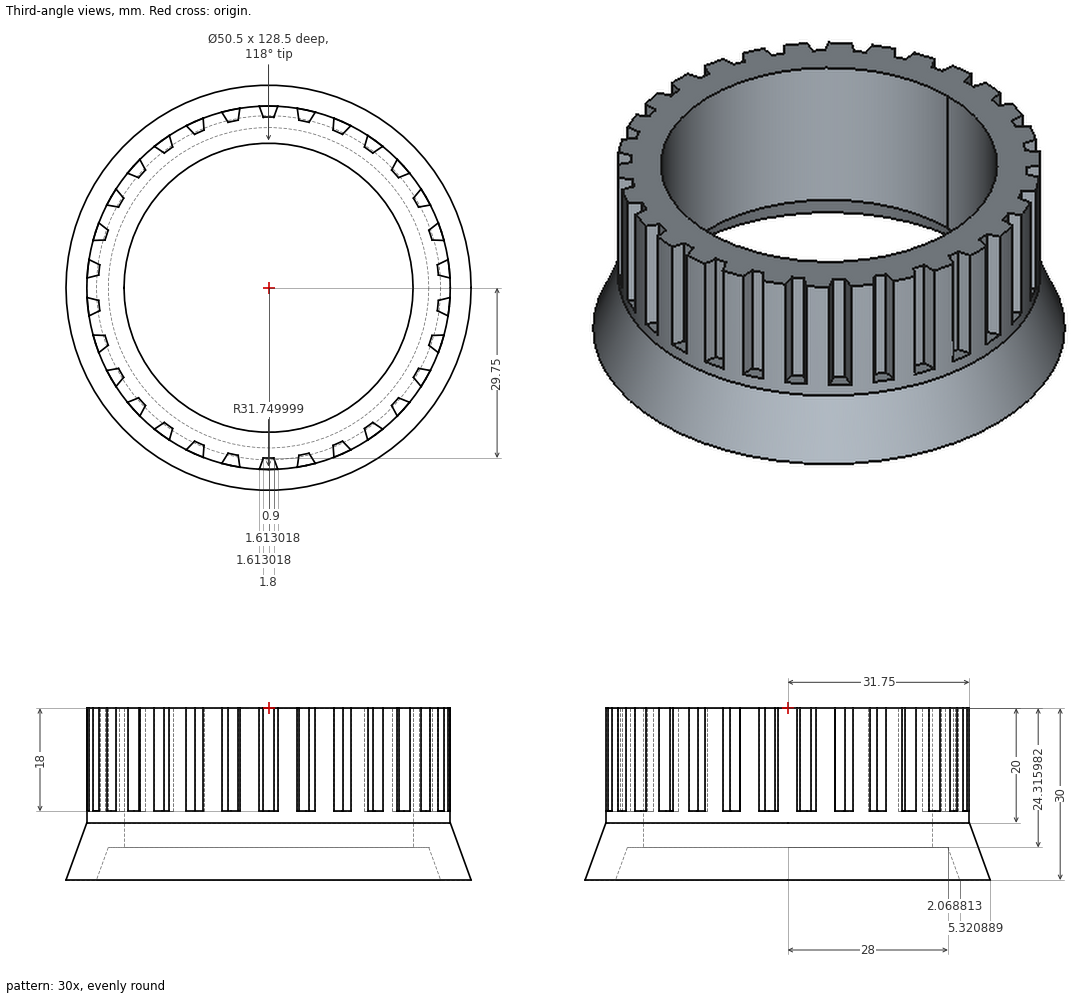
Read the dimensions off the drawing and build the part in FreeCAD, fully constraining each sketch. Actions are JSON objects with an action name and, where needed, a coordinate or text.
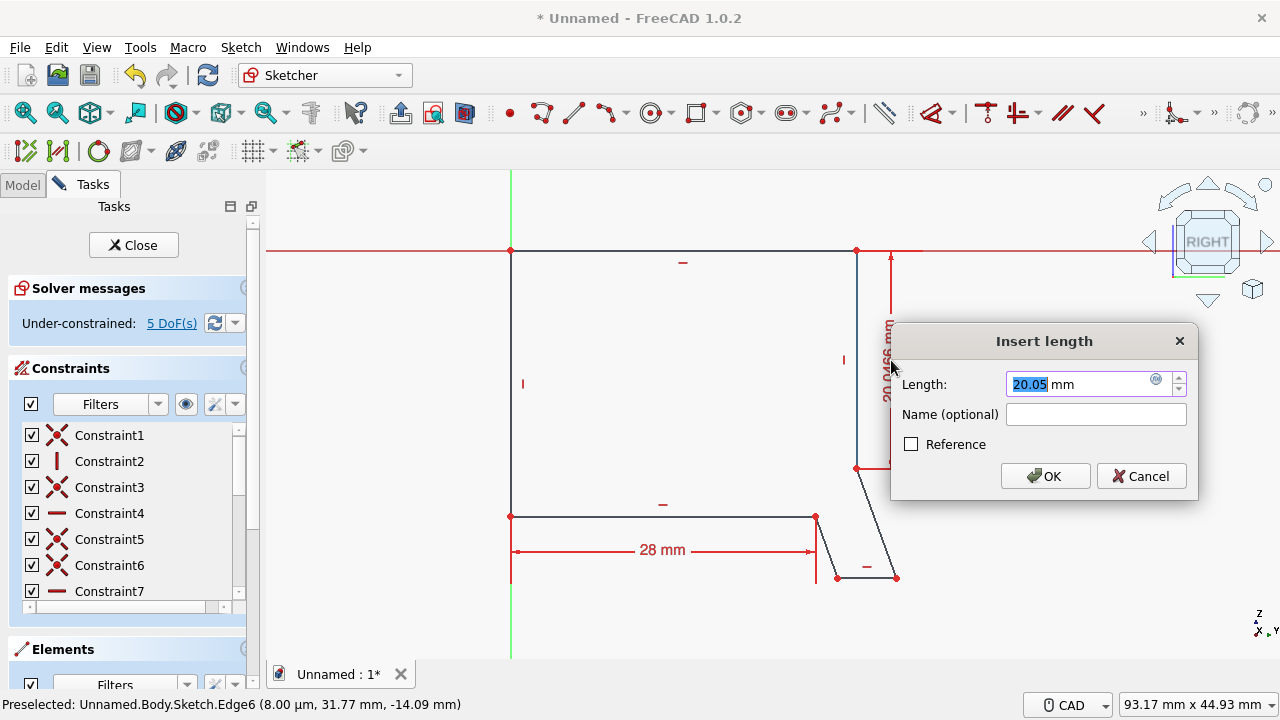
{"action": "type", "text": "20"}
{"action": "key", "text": "Return"}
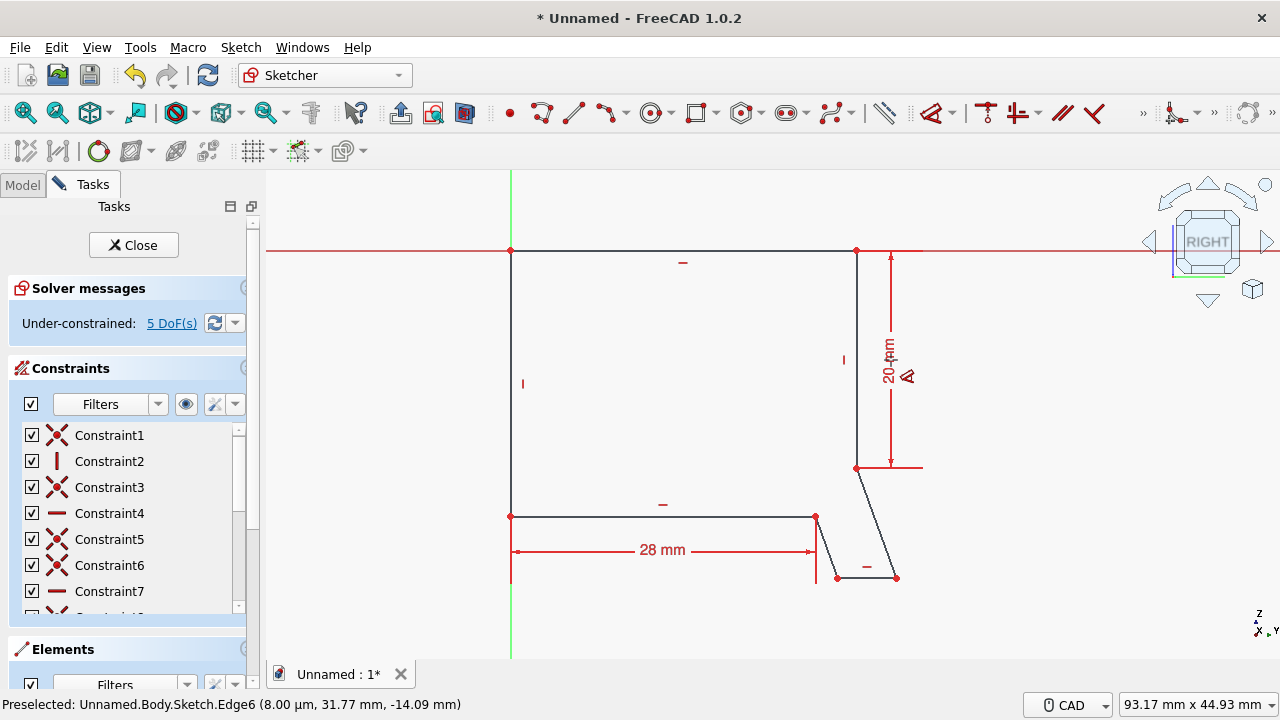
{"action": "left_click", "coordinate": [838, 578]}
{"action": "left_click", "coordinate": [477, 414]}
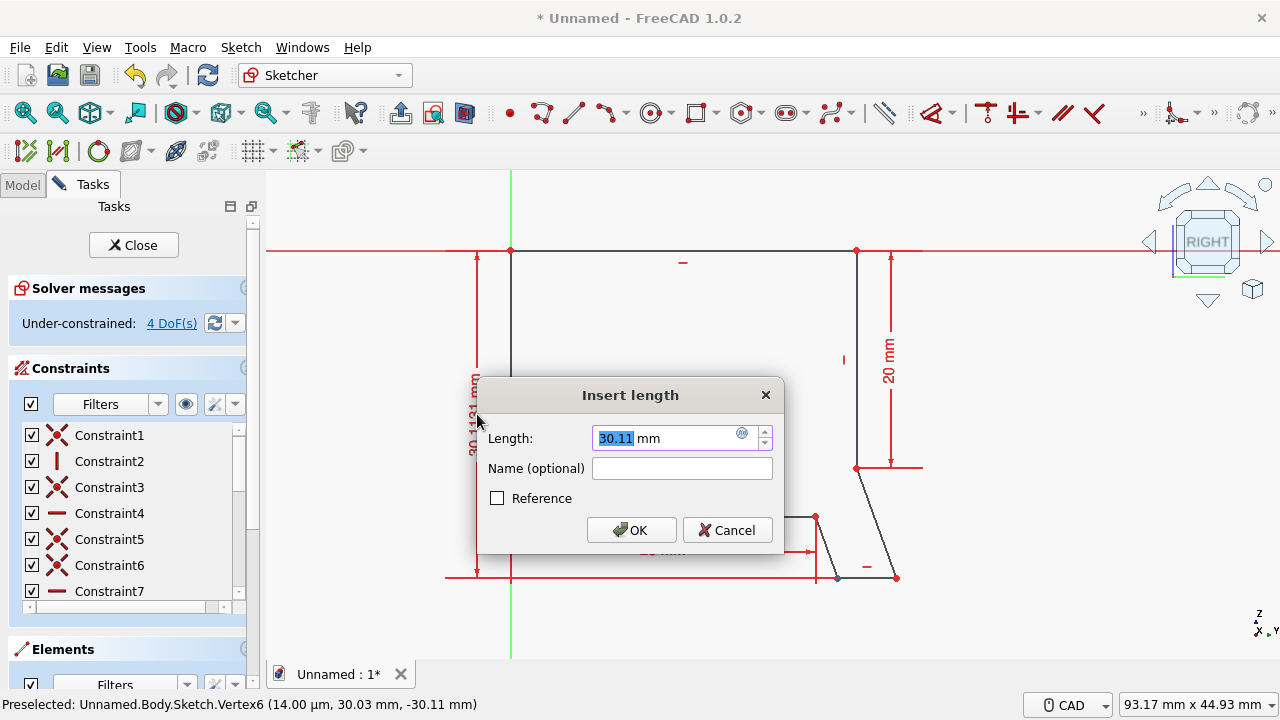
{"action": "type", "text": "30"}
{"action": "key", "text": "Return"}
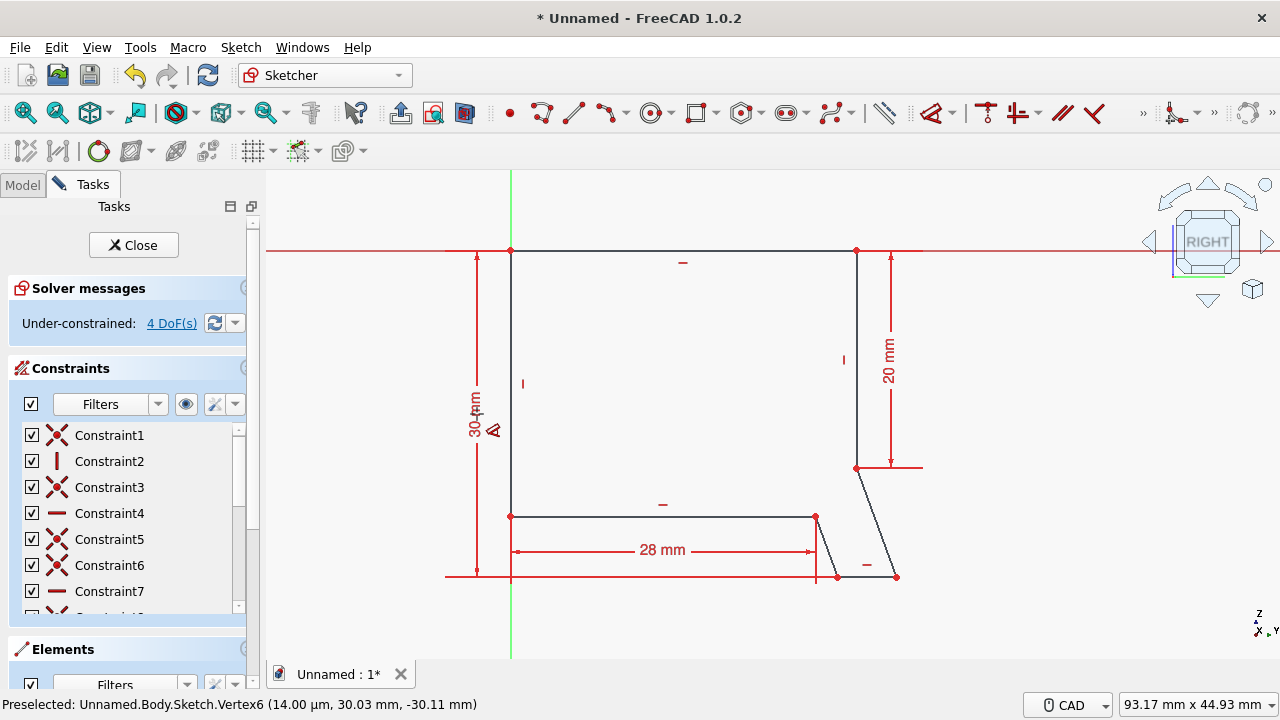
{"action": "left_click", "coordinate": [753, 251]}
{"action": "left_click", "coordinate": [684, 217]}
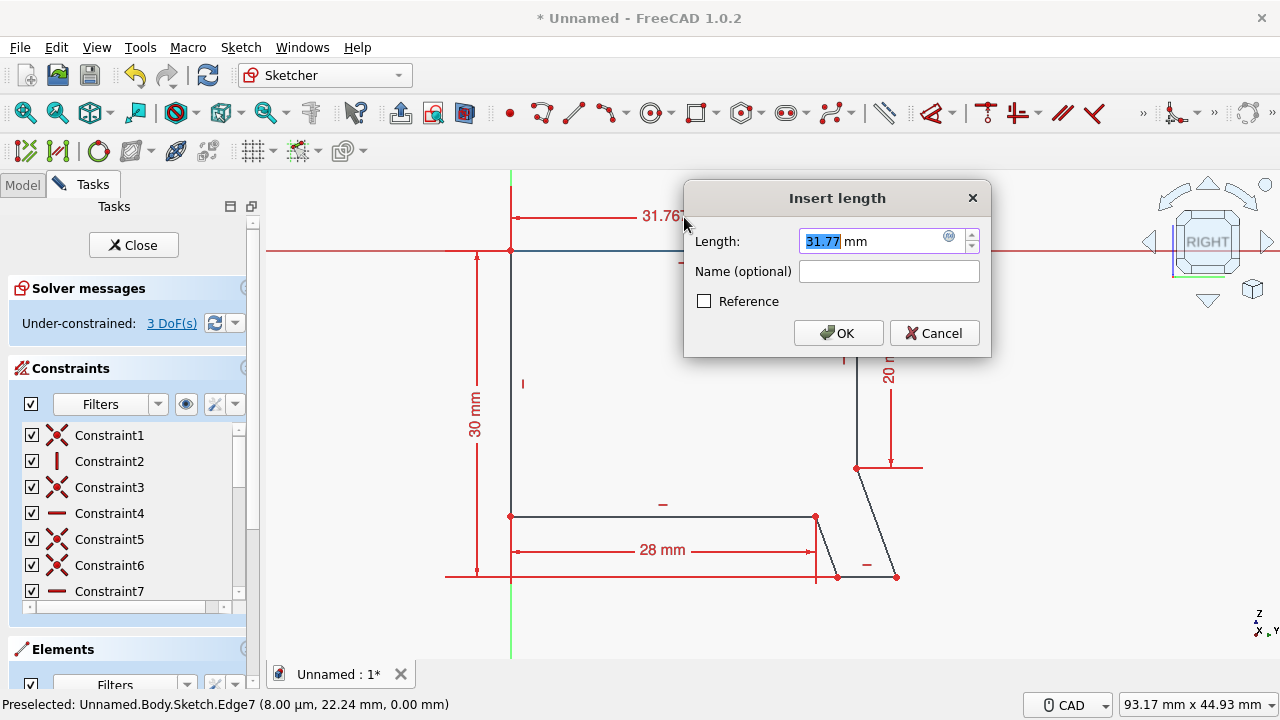
{"action": "type", "text": "31.75"}
{"action": "key", "text": "Return"}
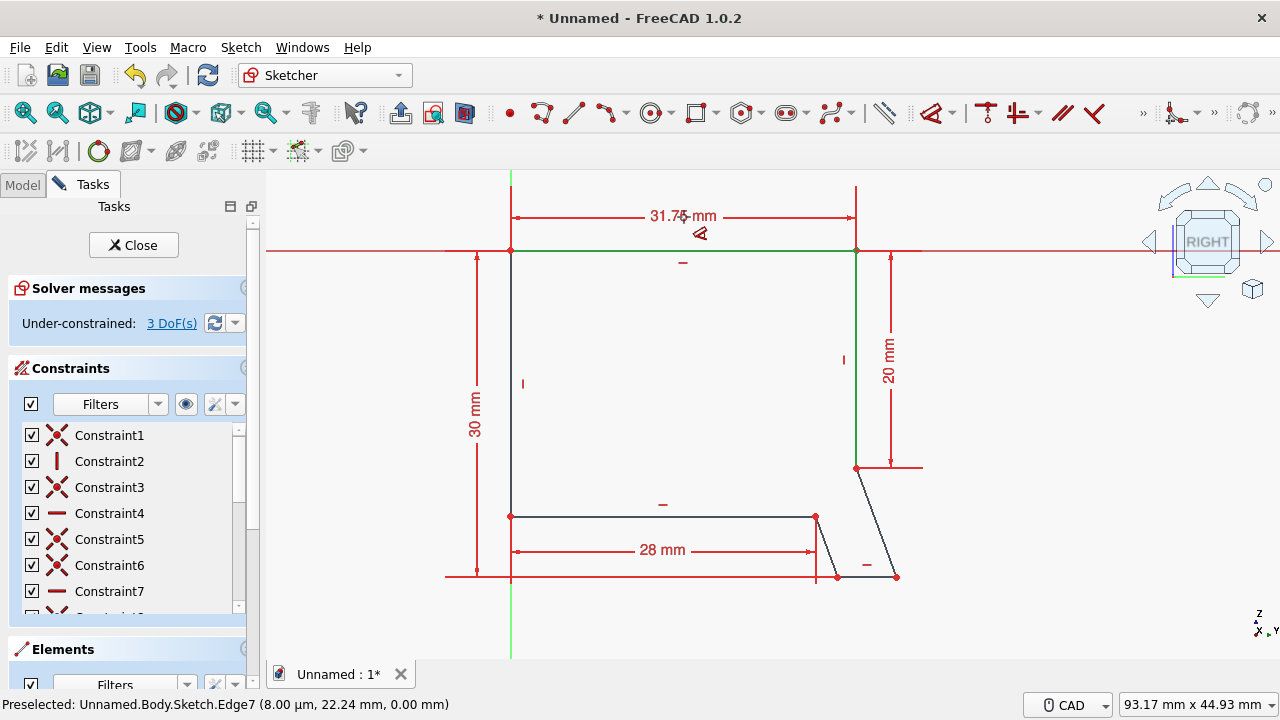
{"action": "left_click", "coordinate": [855, 577]}
{"action": "left_click", "coordinate": [867, 611]}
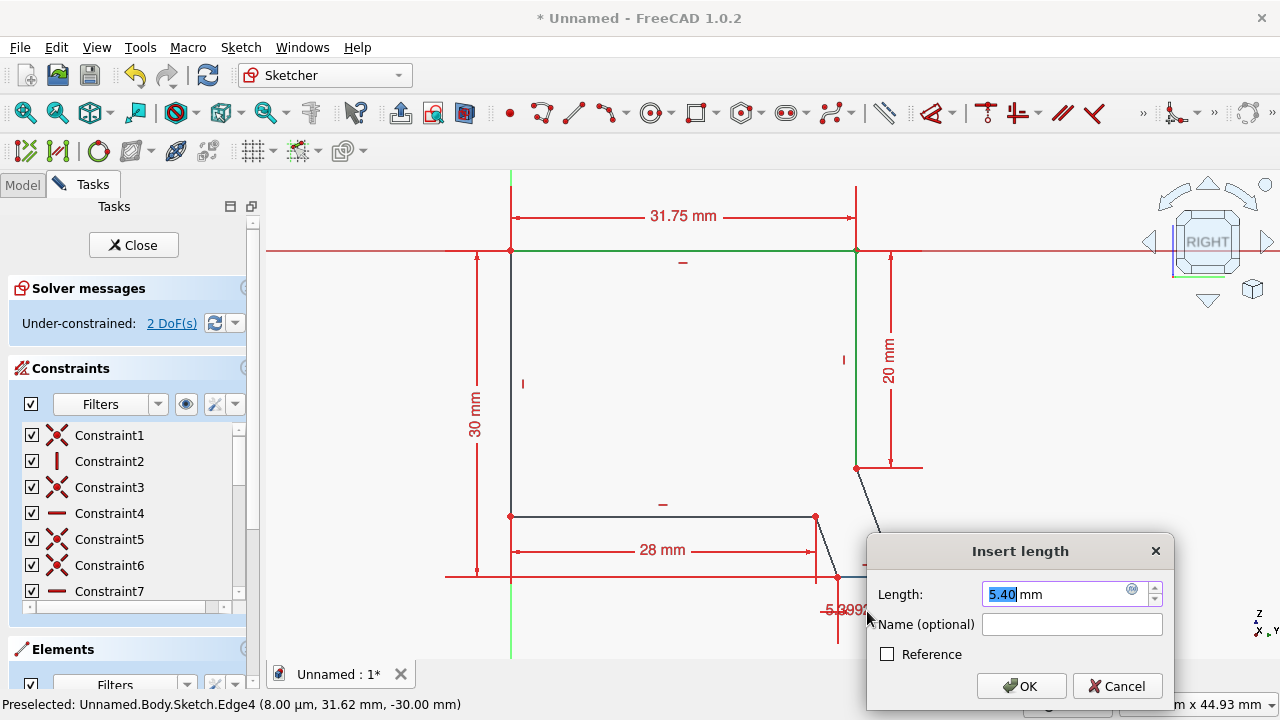
{"action": "type", "text": "5.320889"}
{"action": "key", "text": "Return"}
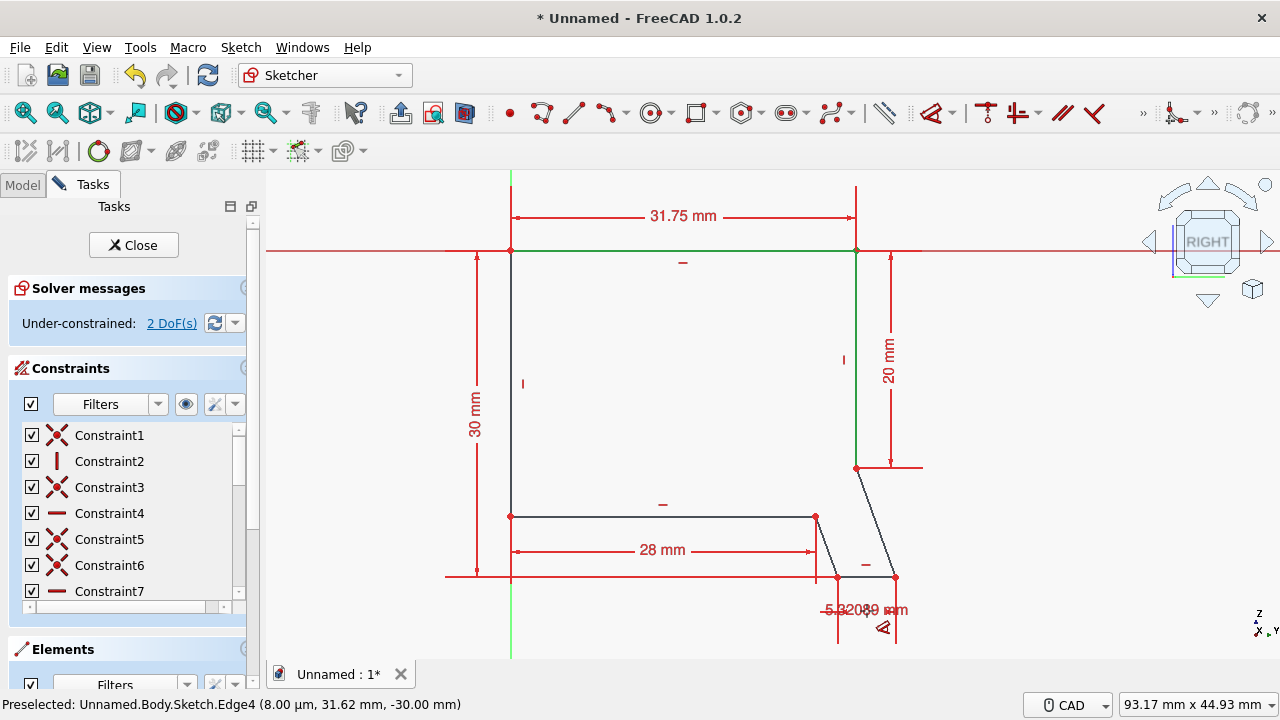
{"action": "left_click", "coordinate": [511, 330]}
{"action": "left_click", "coordinate": [477, 384]}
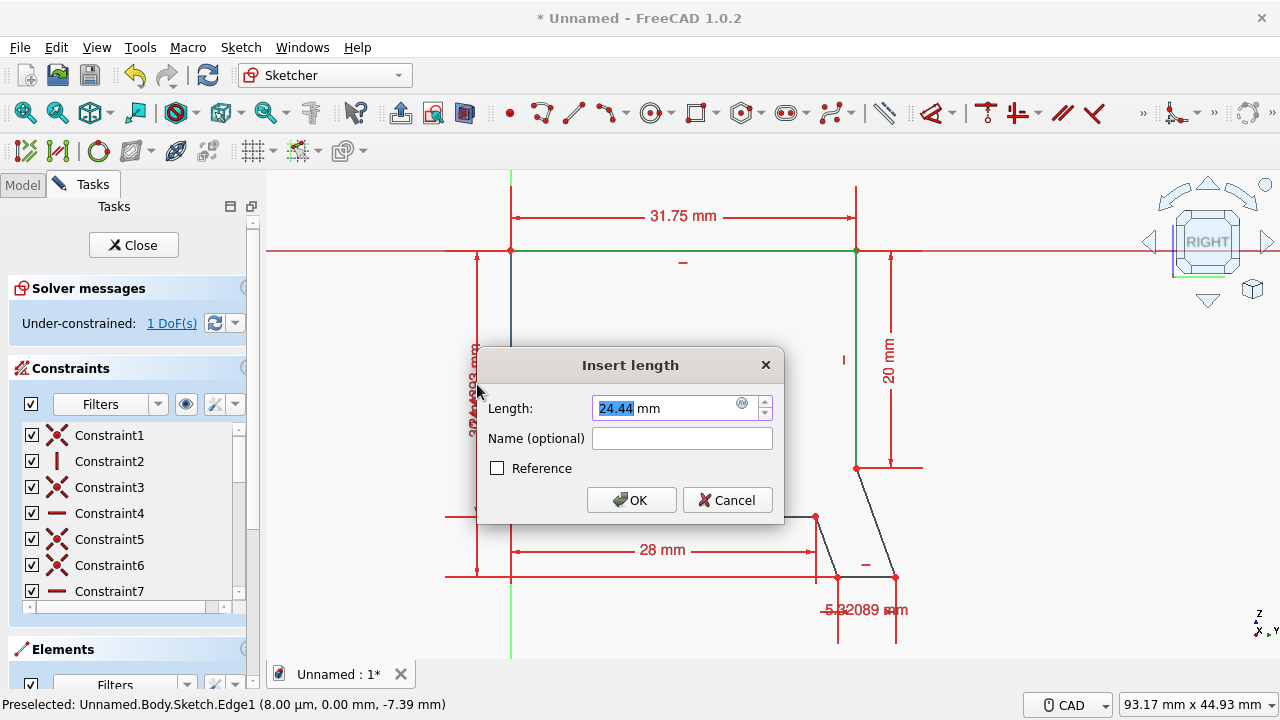
{"action": "type", "text": "24.315982"}
{"action": "key", "text": "Return"}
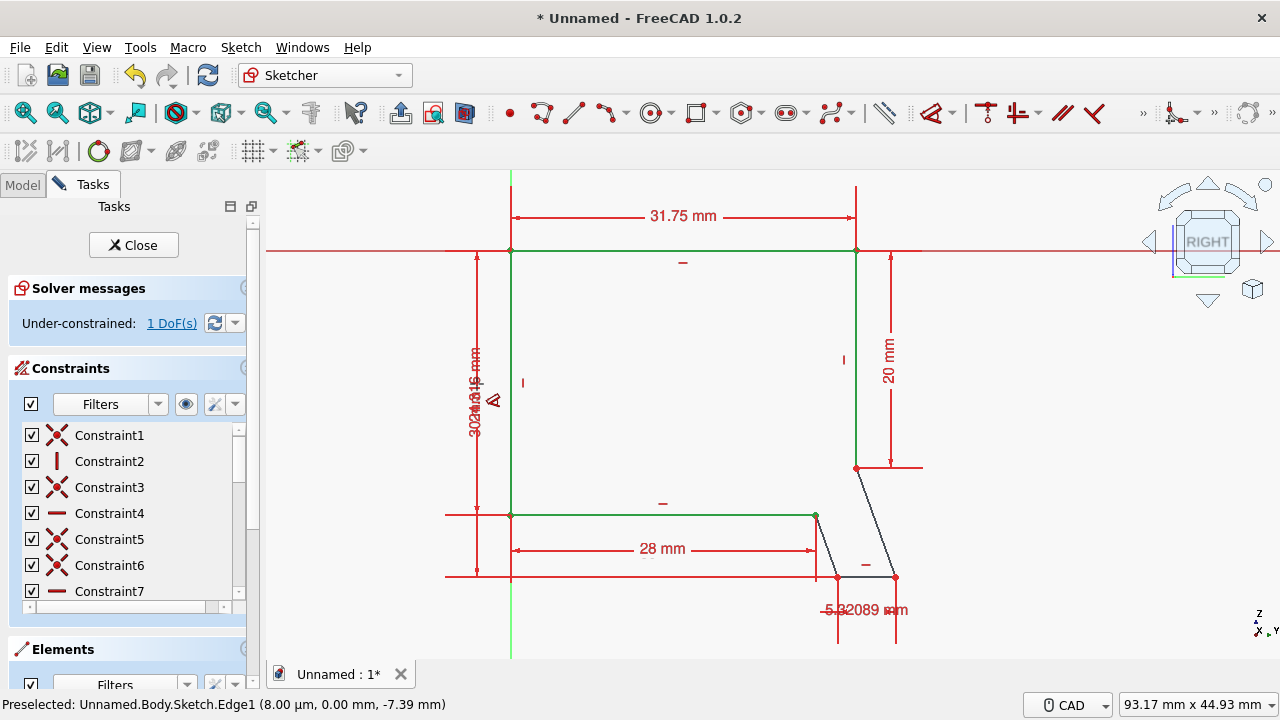
{"action": "scroll", "coordinate": [822, 534], "scroll_direction": "up", "scroll_amount": 3}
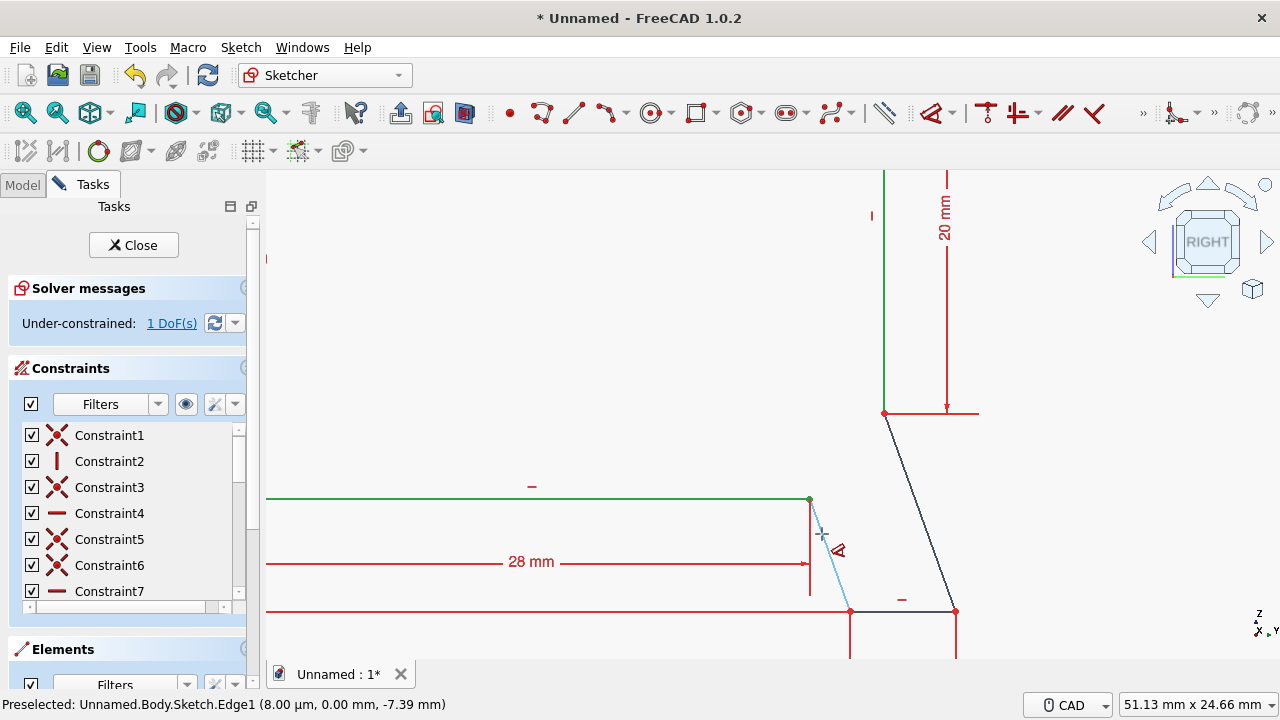
{"action": "left_click", "coordinate": [822, 533]}
{"action": "left_click", "coordinate": [830, 465]}